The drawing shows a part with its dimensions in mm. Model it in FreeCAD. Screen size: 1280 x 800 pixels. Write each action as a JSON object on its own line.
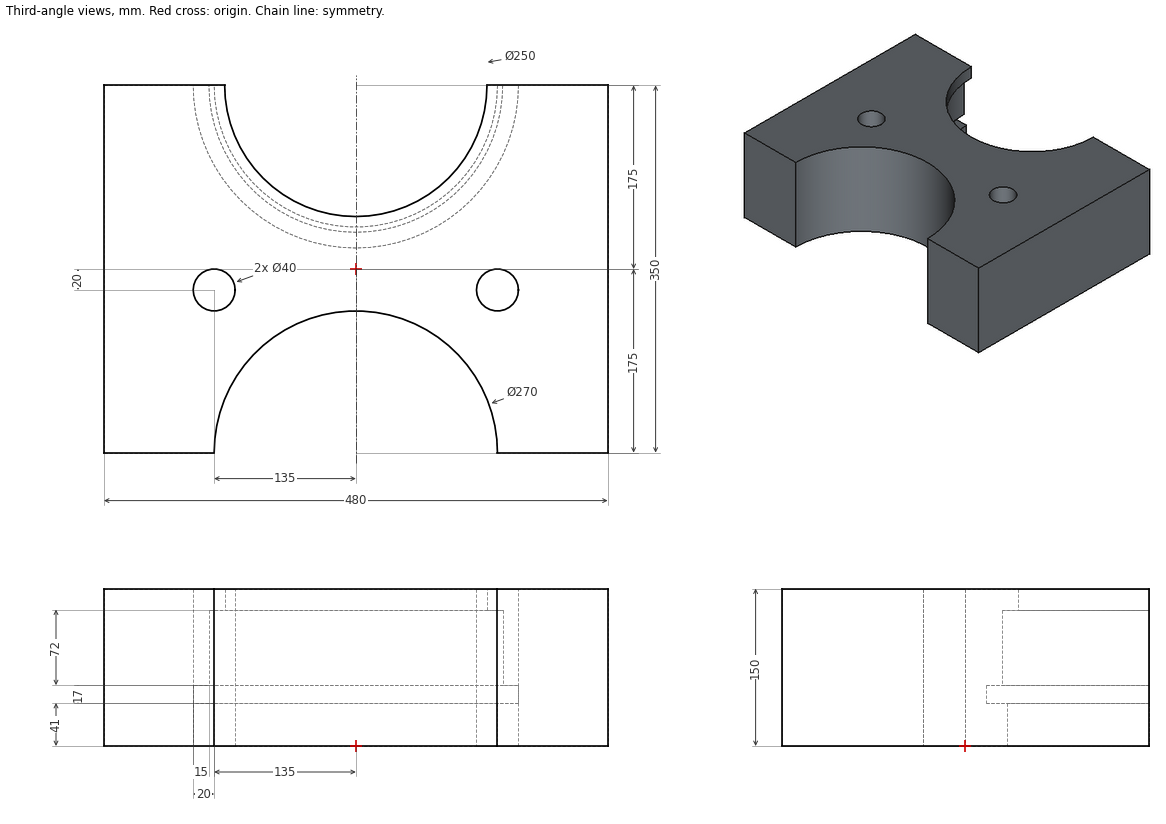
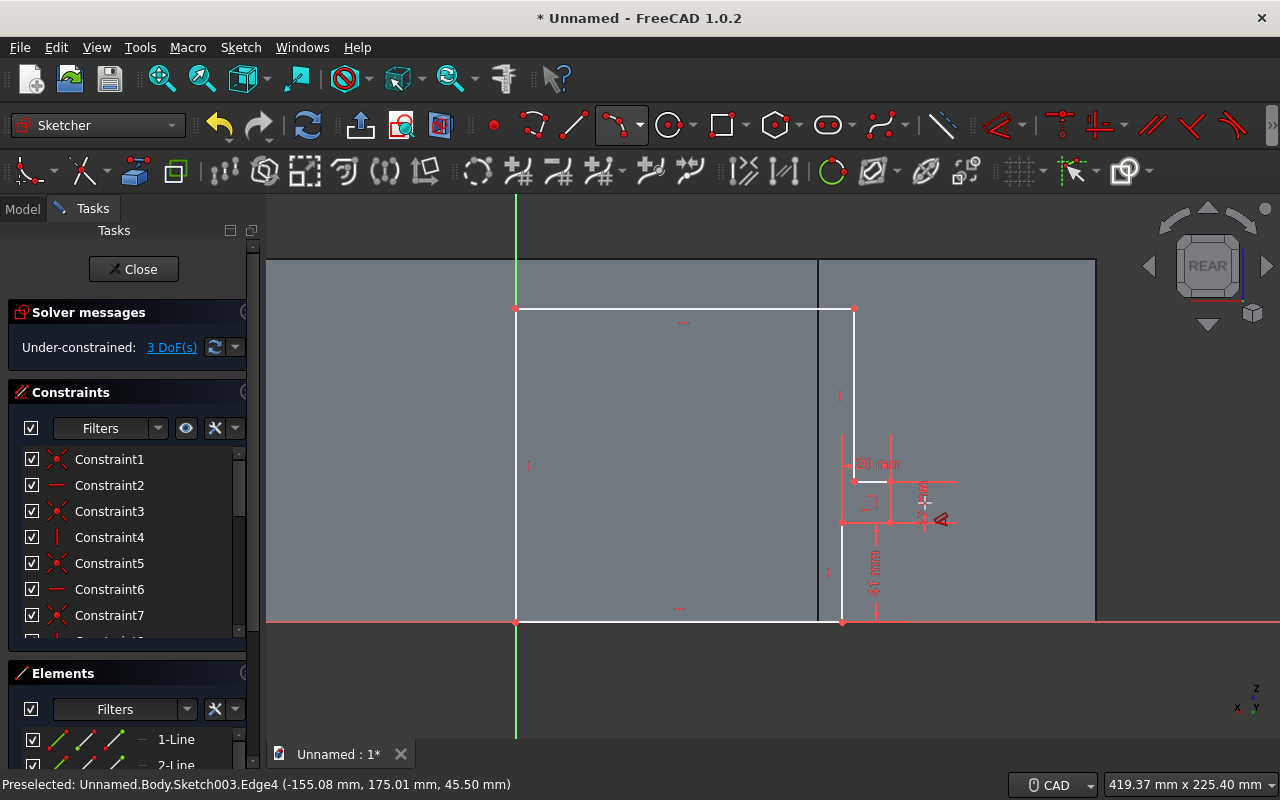
{"action": "scroll", "coordinate": [880, 482], "scroll_direction": "up", "scroll_amount": 2}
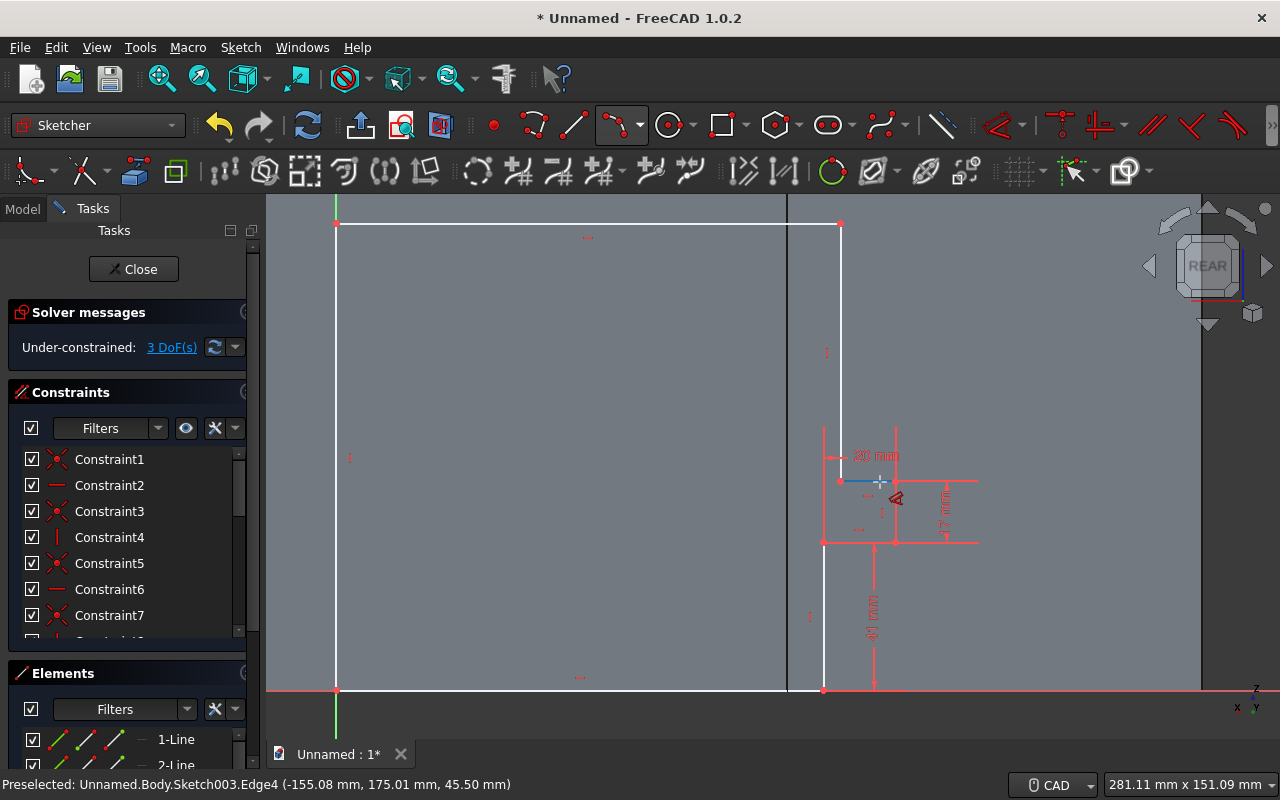
{"action": "left_click", "coordinate": [879, 481]}
{"action": "left_click", "coordinate": [868, 515]}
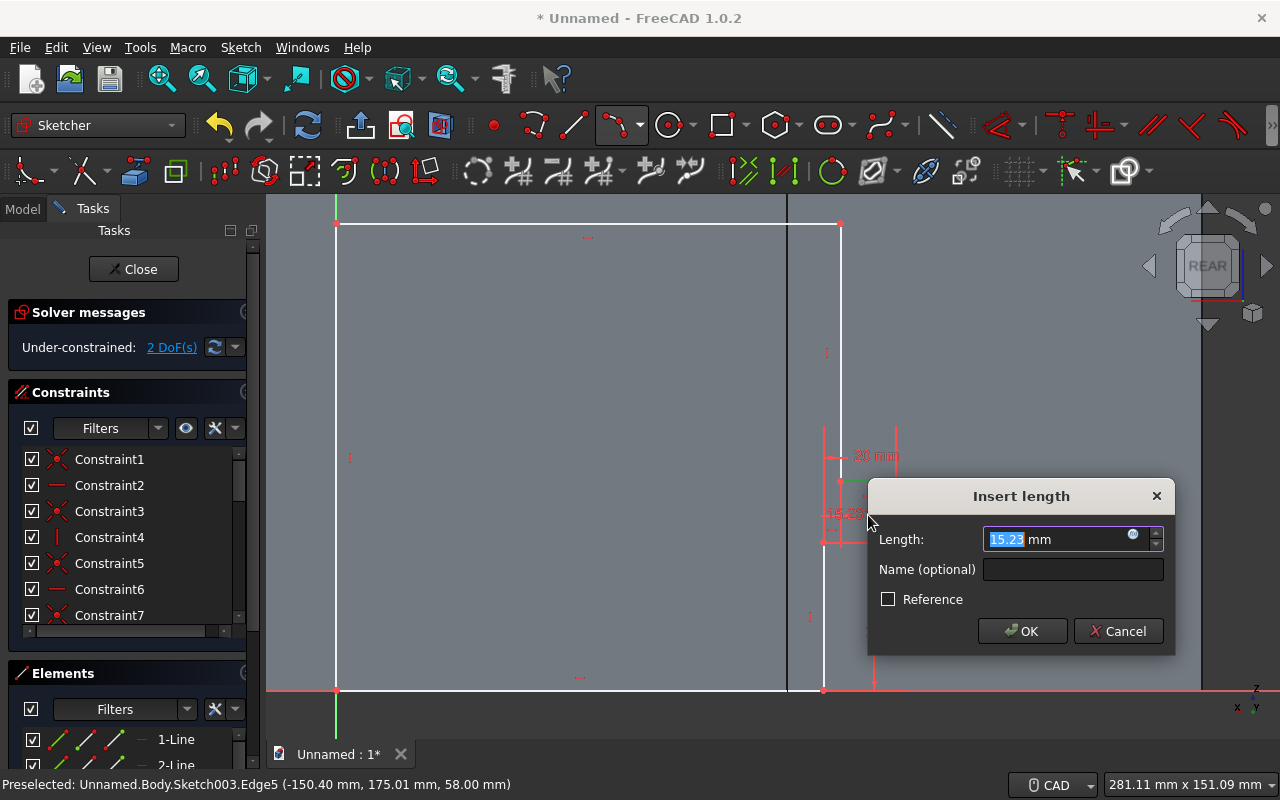
{"action": "type", "text": "15"}
{"action": "key", "text": "Return"}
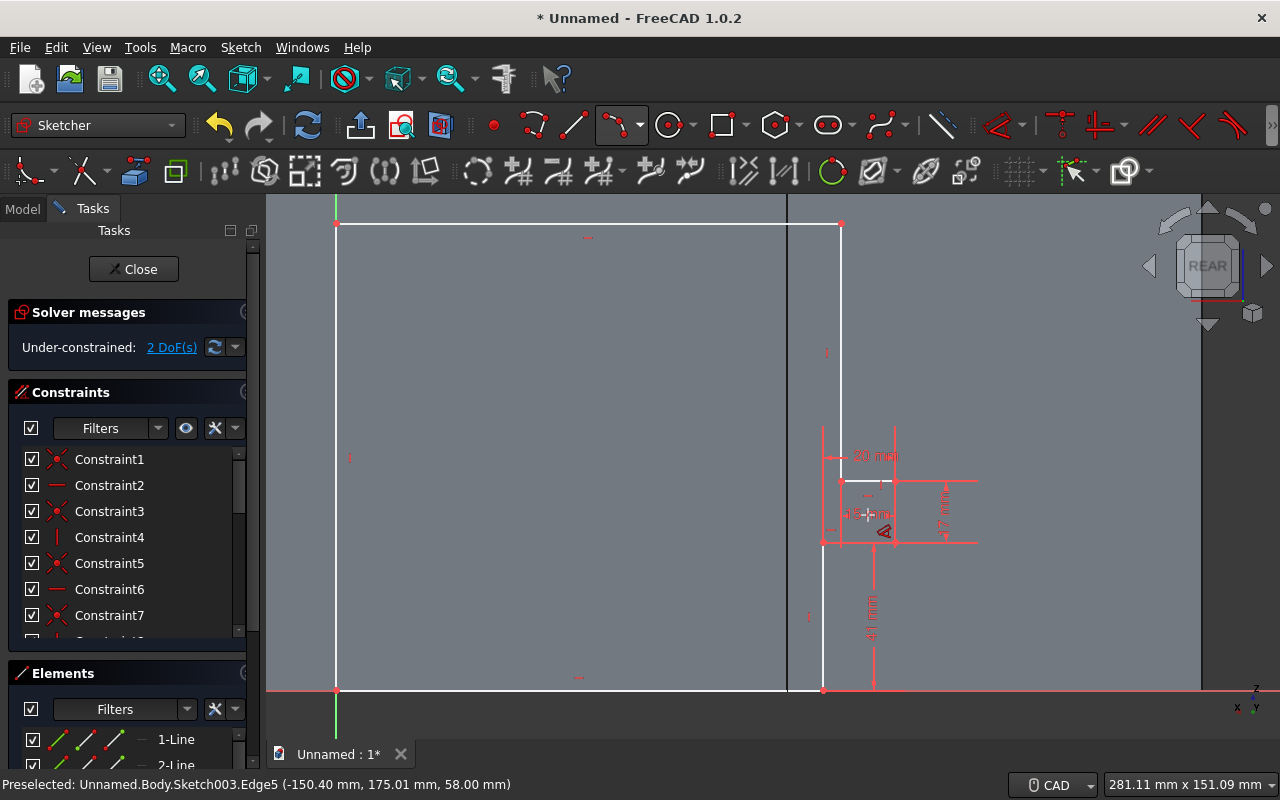
{"action": "left_click", "coordinate": [841, 404]}
{"action": "left_click", "coordinate": [875, 353]}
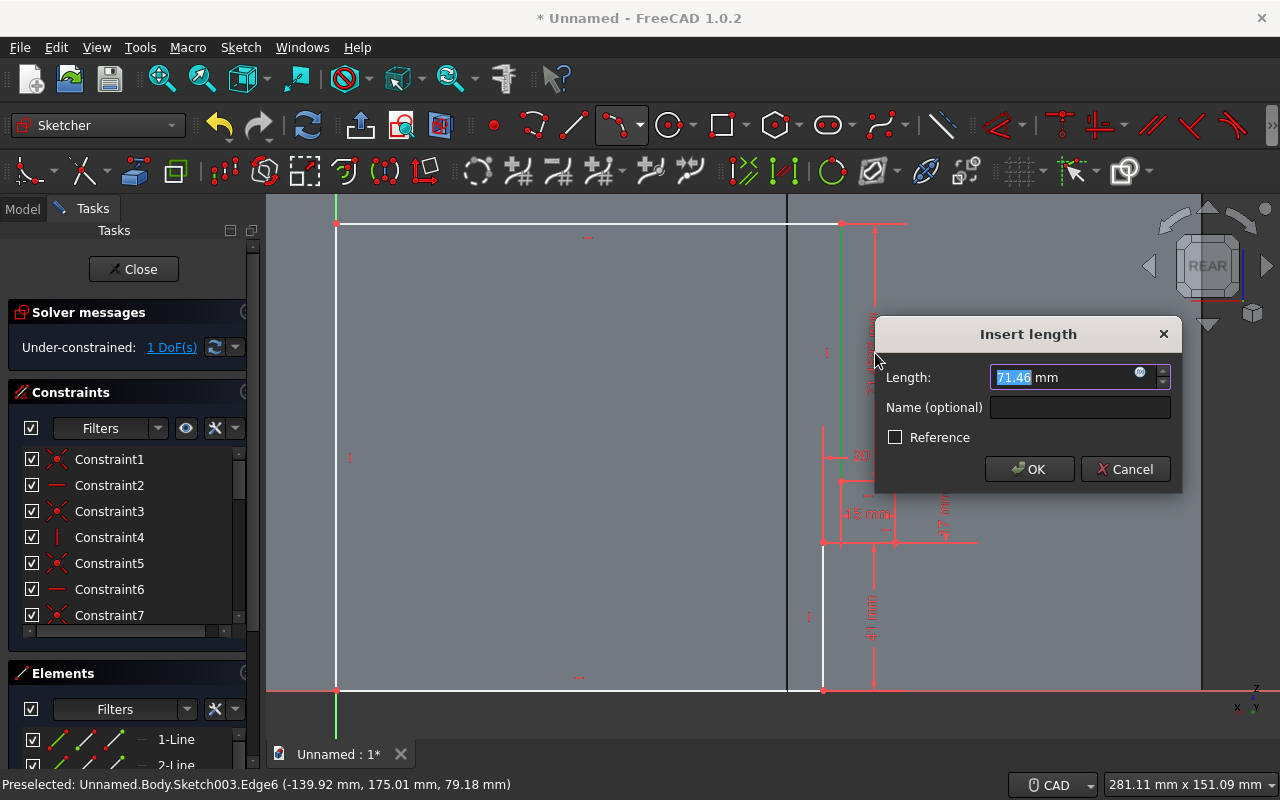
{"action": "type", "text": "72"}
{"action": "key", "text": "Return"}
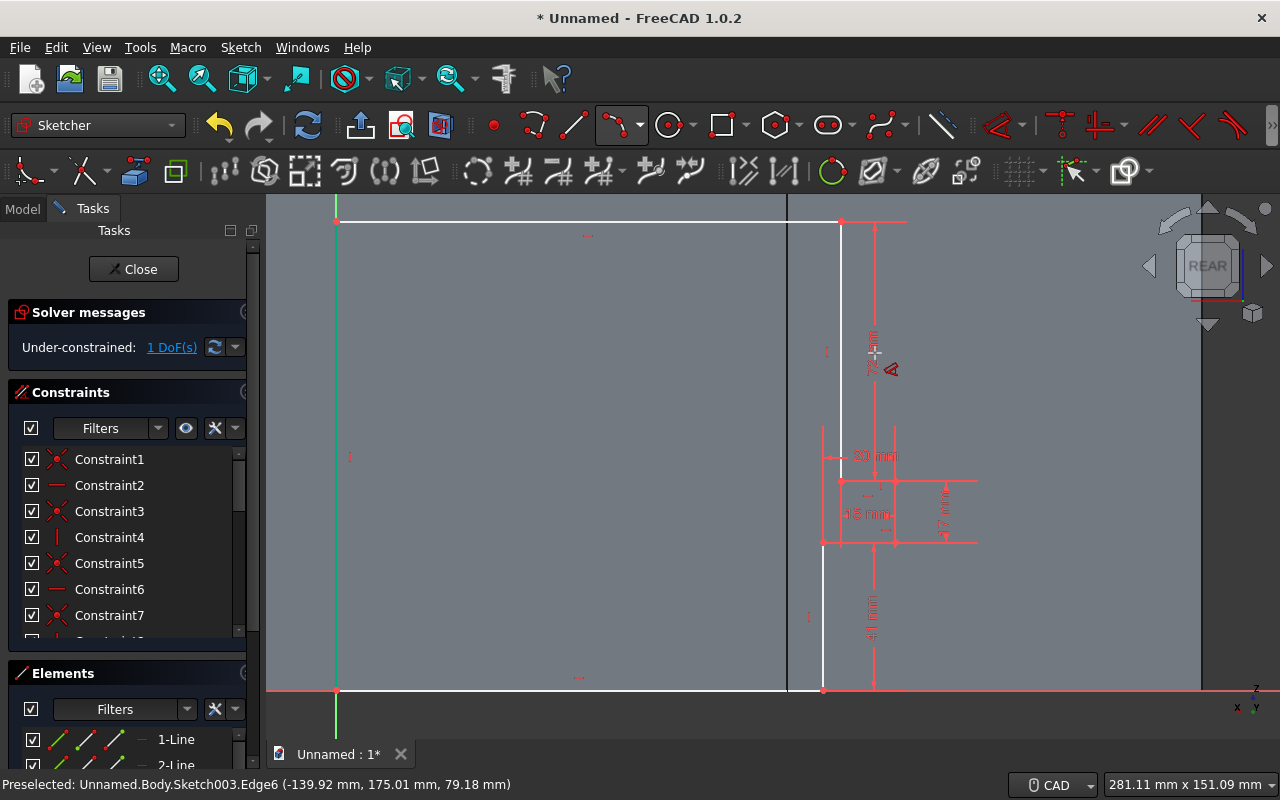
{"action": "left_click", "coordinate": [482, 691]}
{"action": "left_click", "coordinate": [580, 657]}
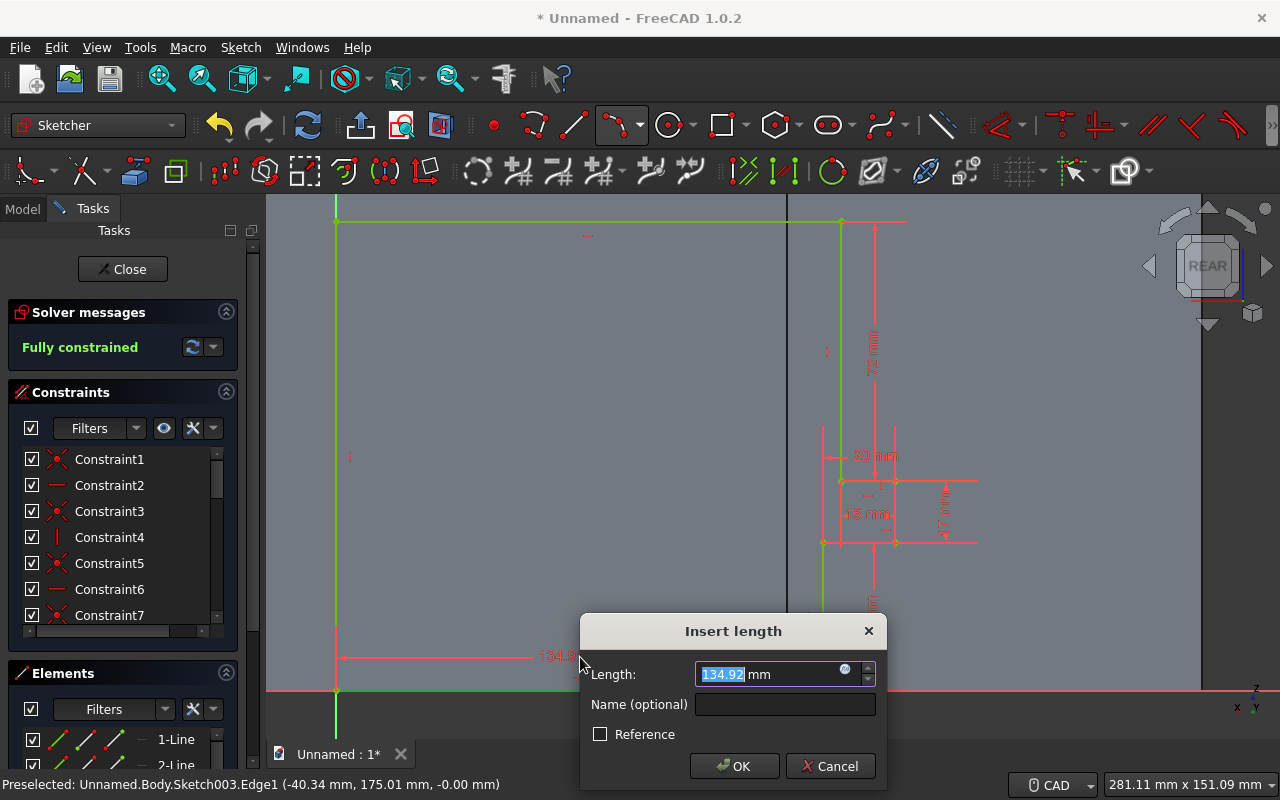
{"action": "type", "text": "135"}
{"action": "key", "text": "Return"}
{"action": "key", "text": "Escape"}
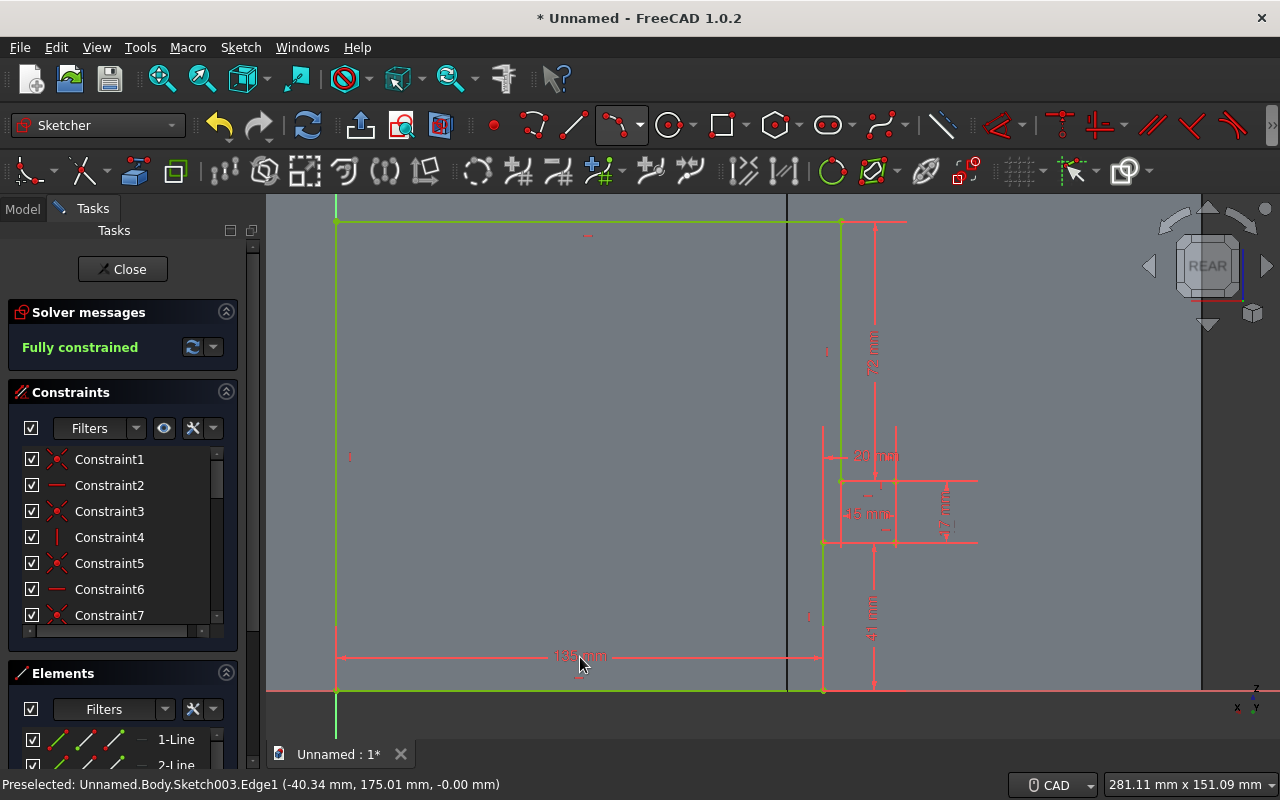
{"action": "left_click", "coordinate": [123, 269]}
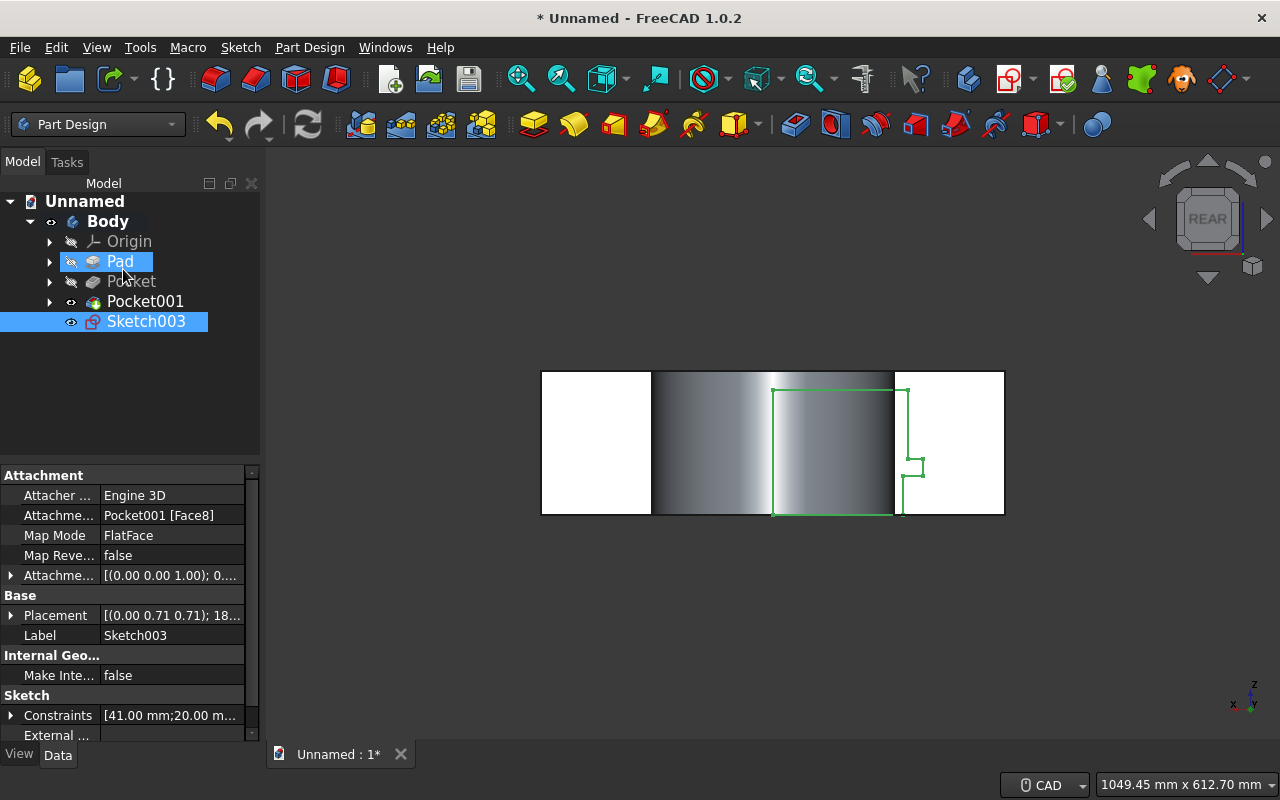
{"action": "left_click", "coordinate": [876, 124]}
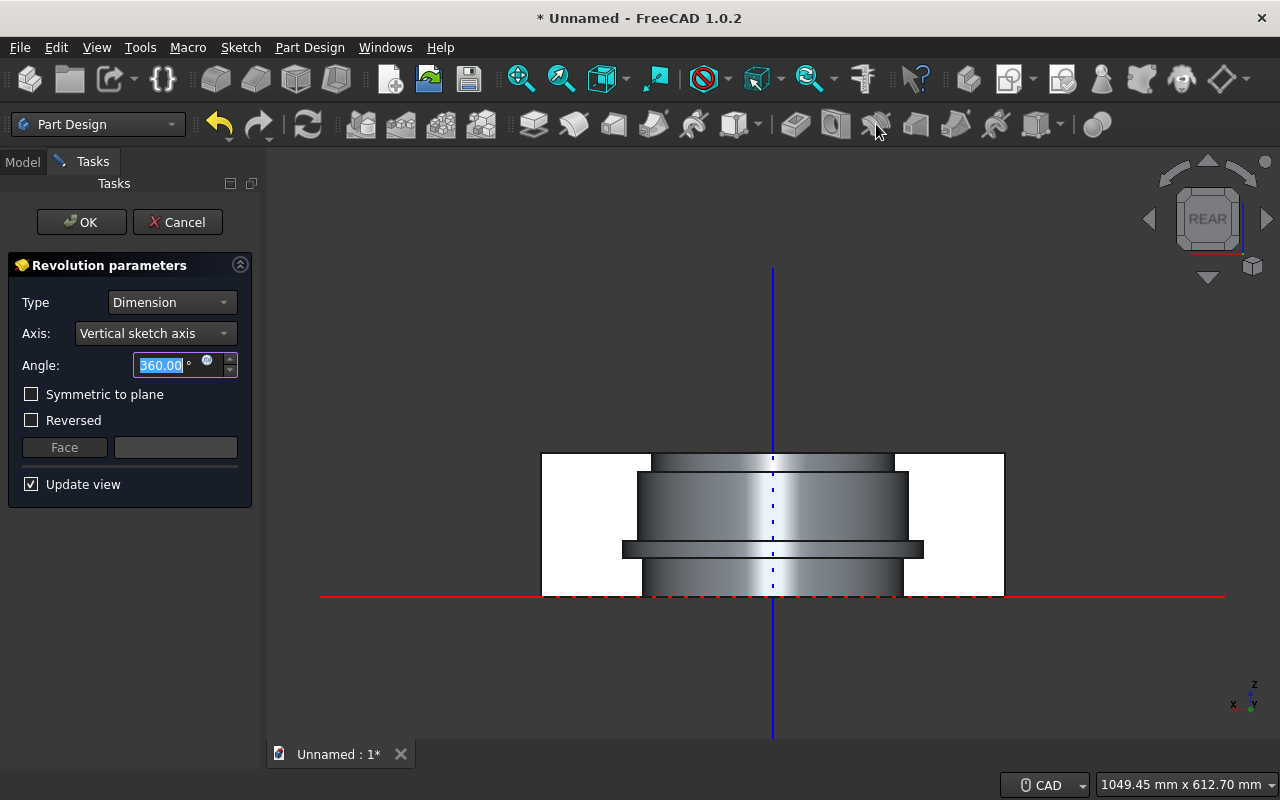
{"action": "left_click", "coordinate": [82, 222]}